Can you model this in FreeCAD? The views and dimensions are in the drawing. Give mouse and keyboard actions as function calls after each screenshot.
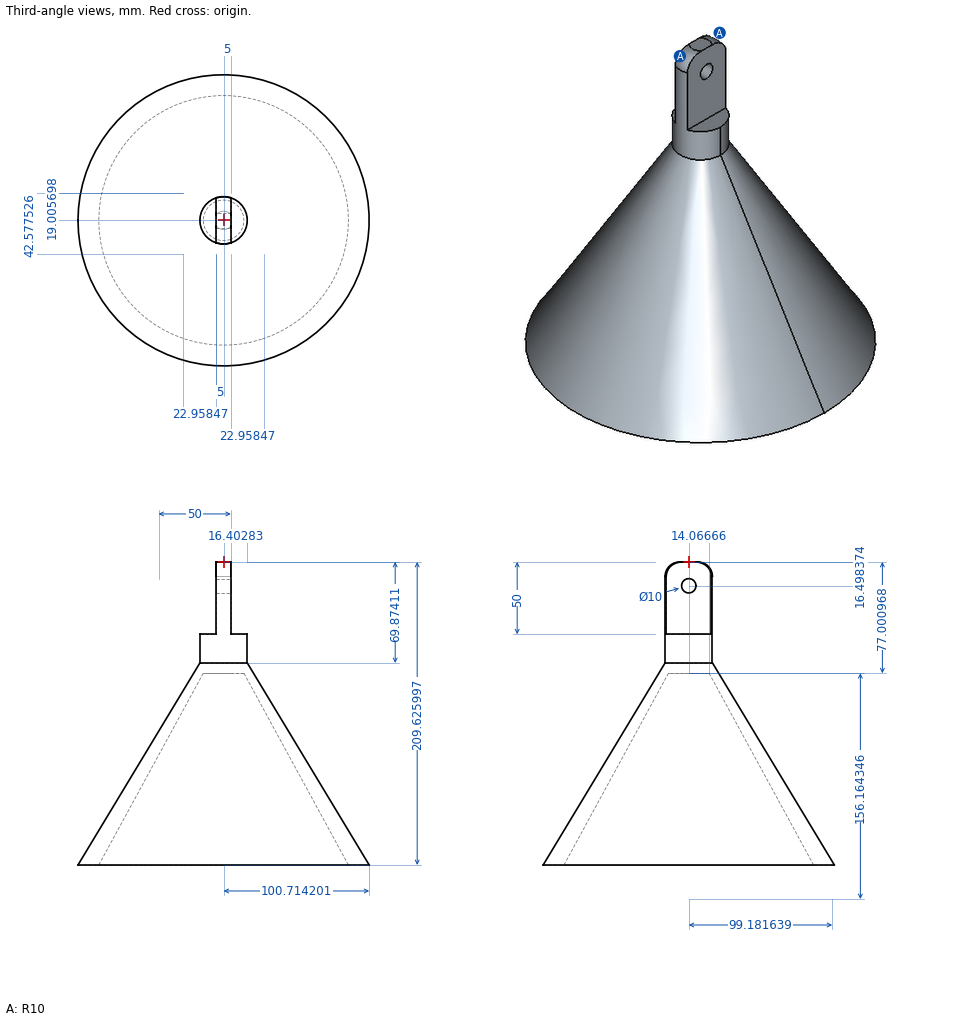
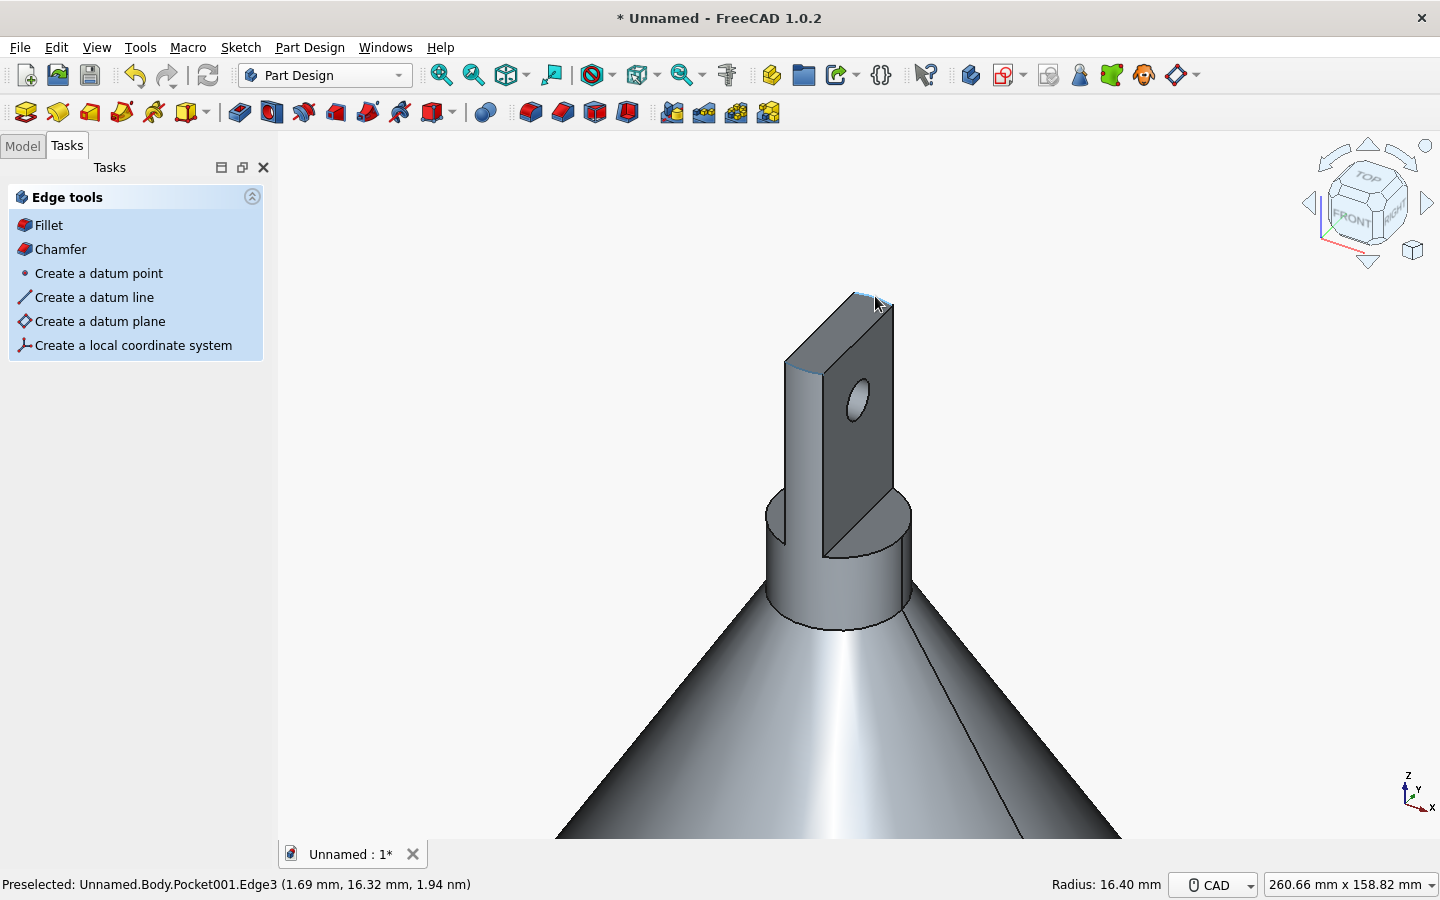
click(442, 76)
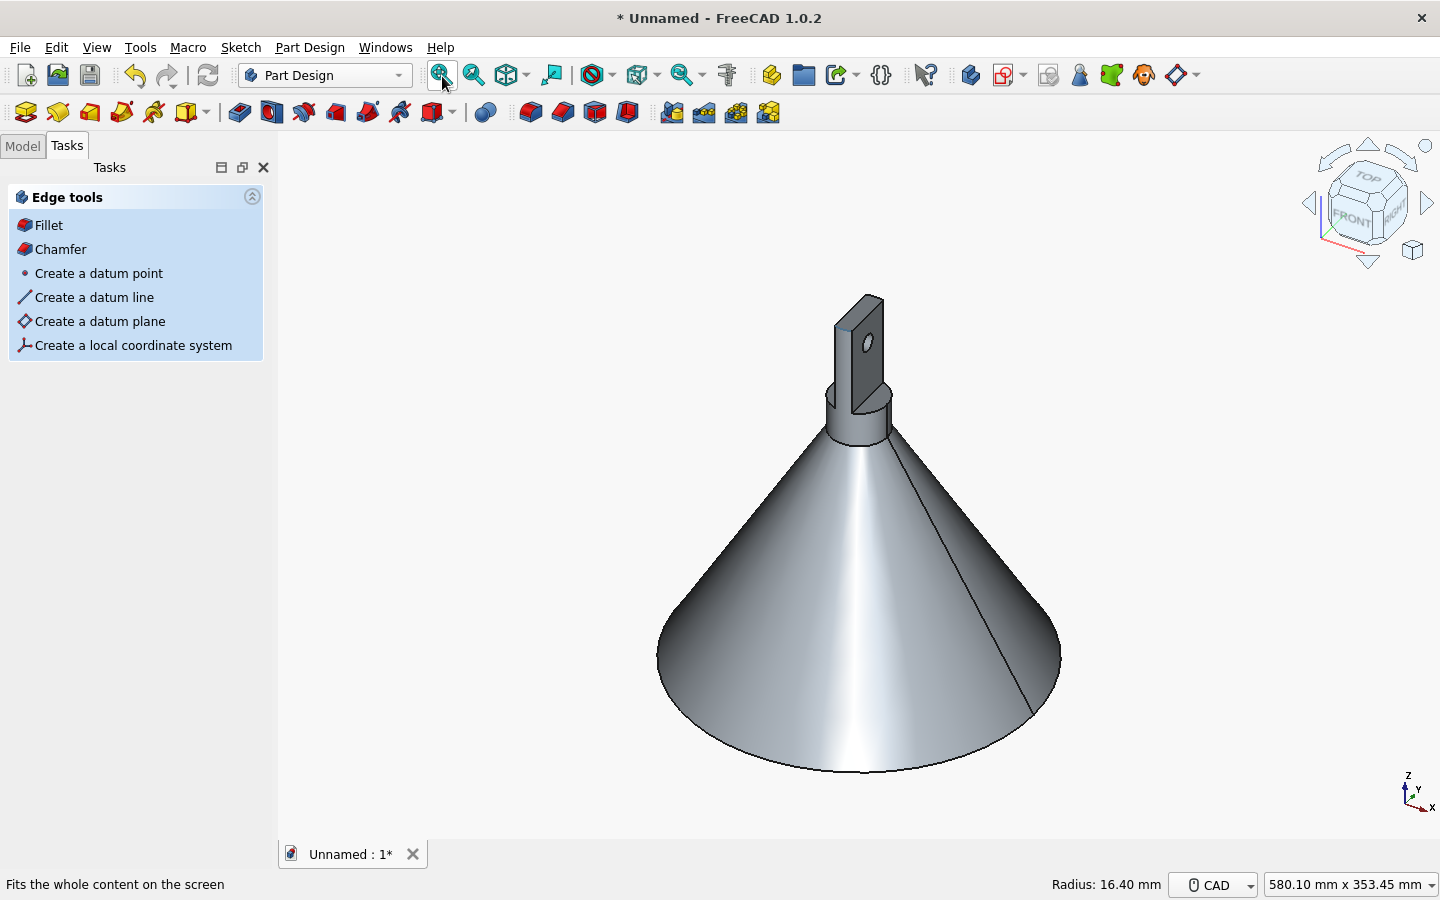
key(0)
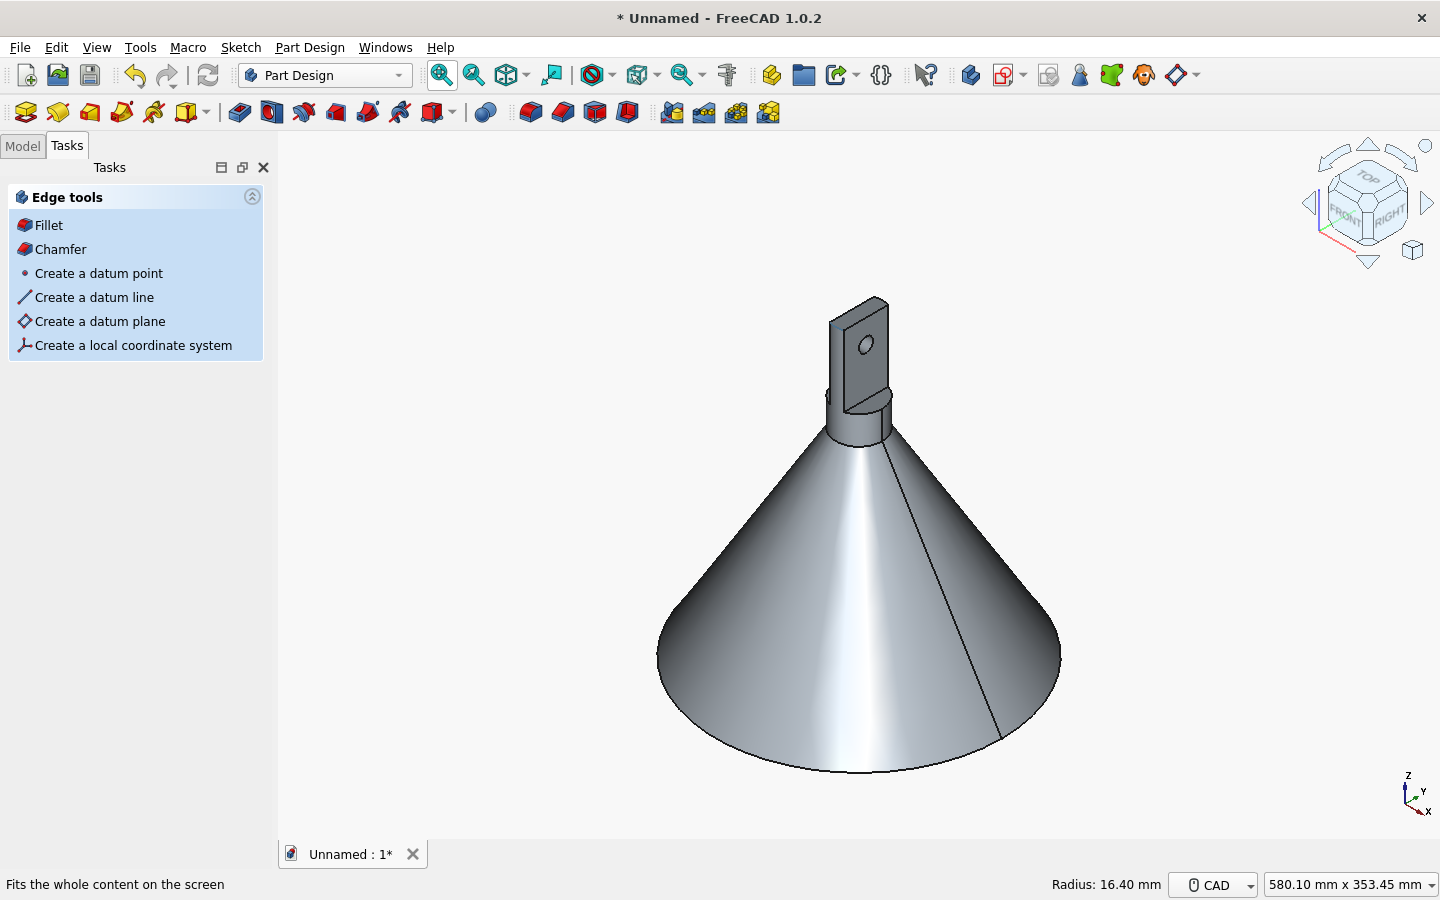
click(882, 299, ctrl)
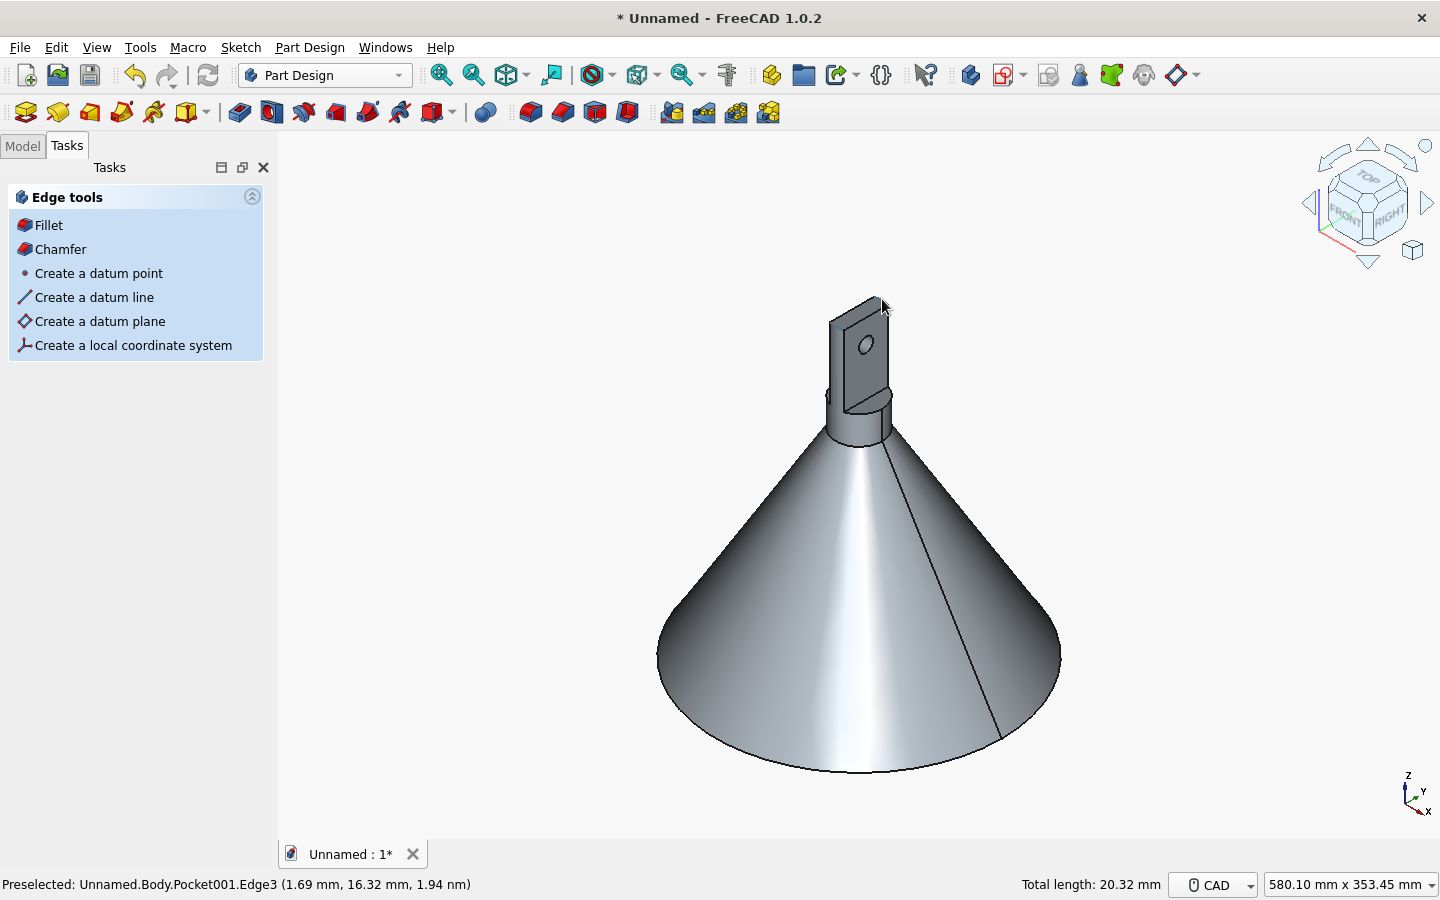
click(532, 112)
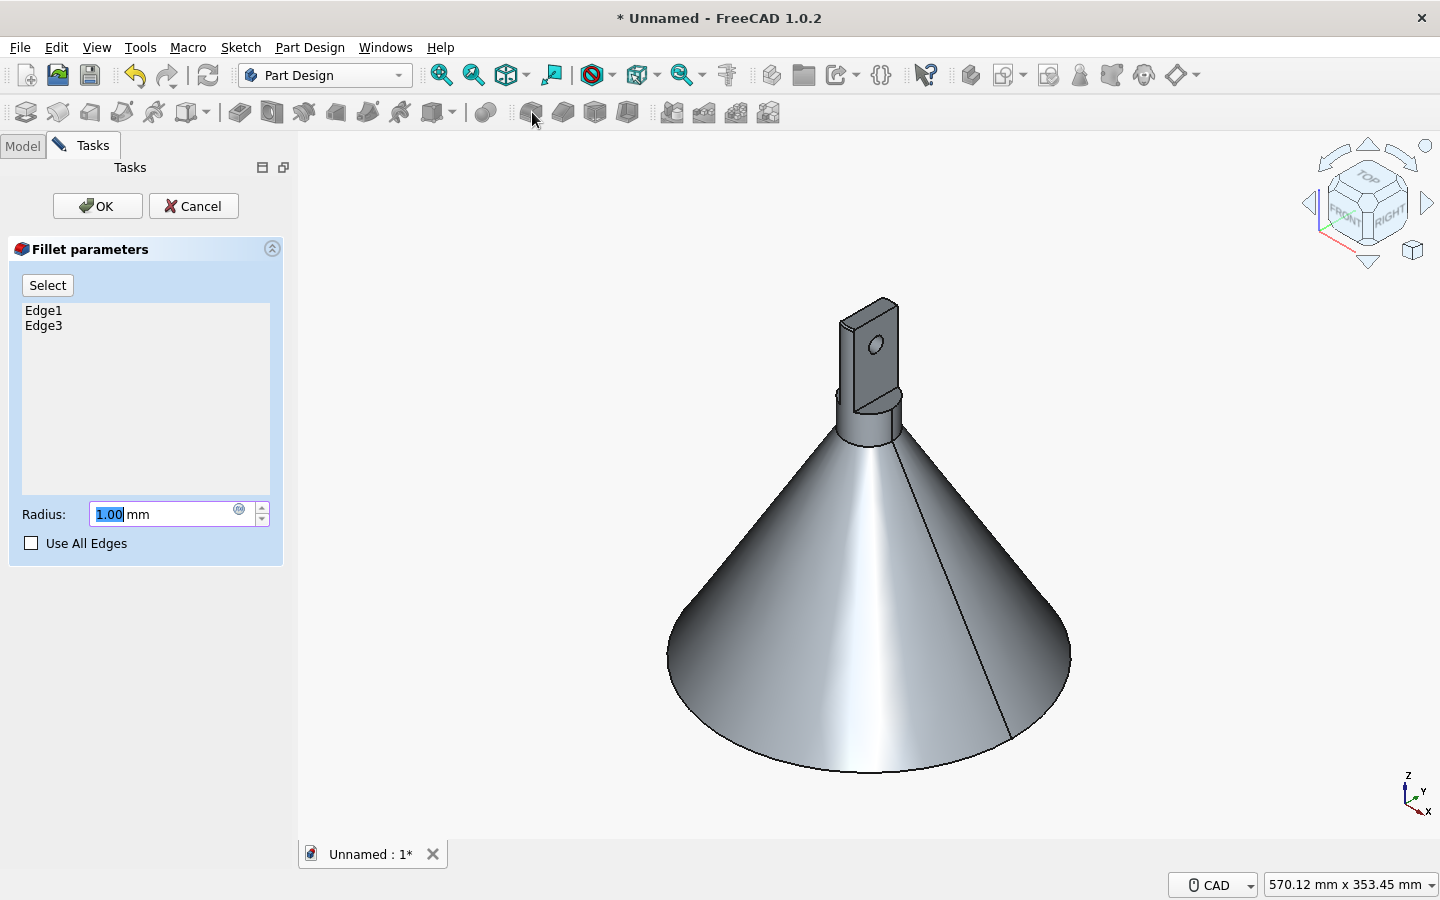
text(10)
key(Tab)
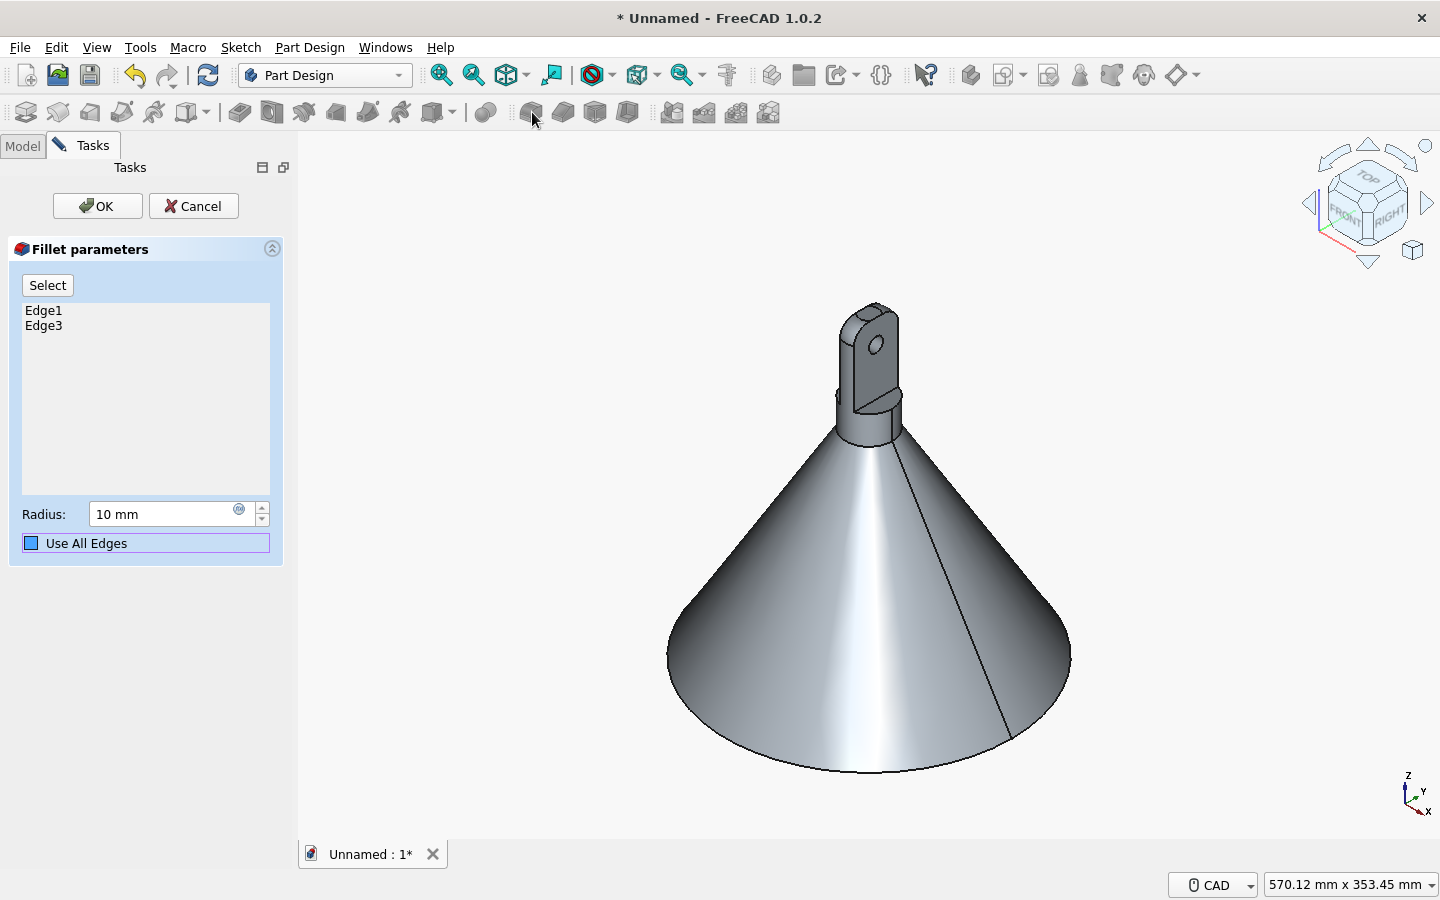
click(98, 206)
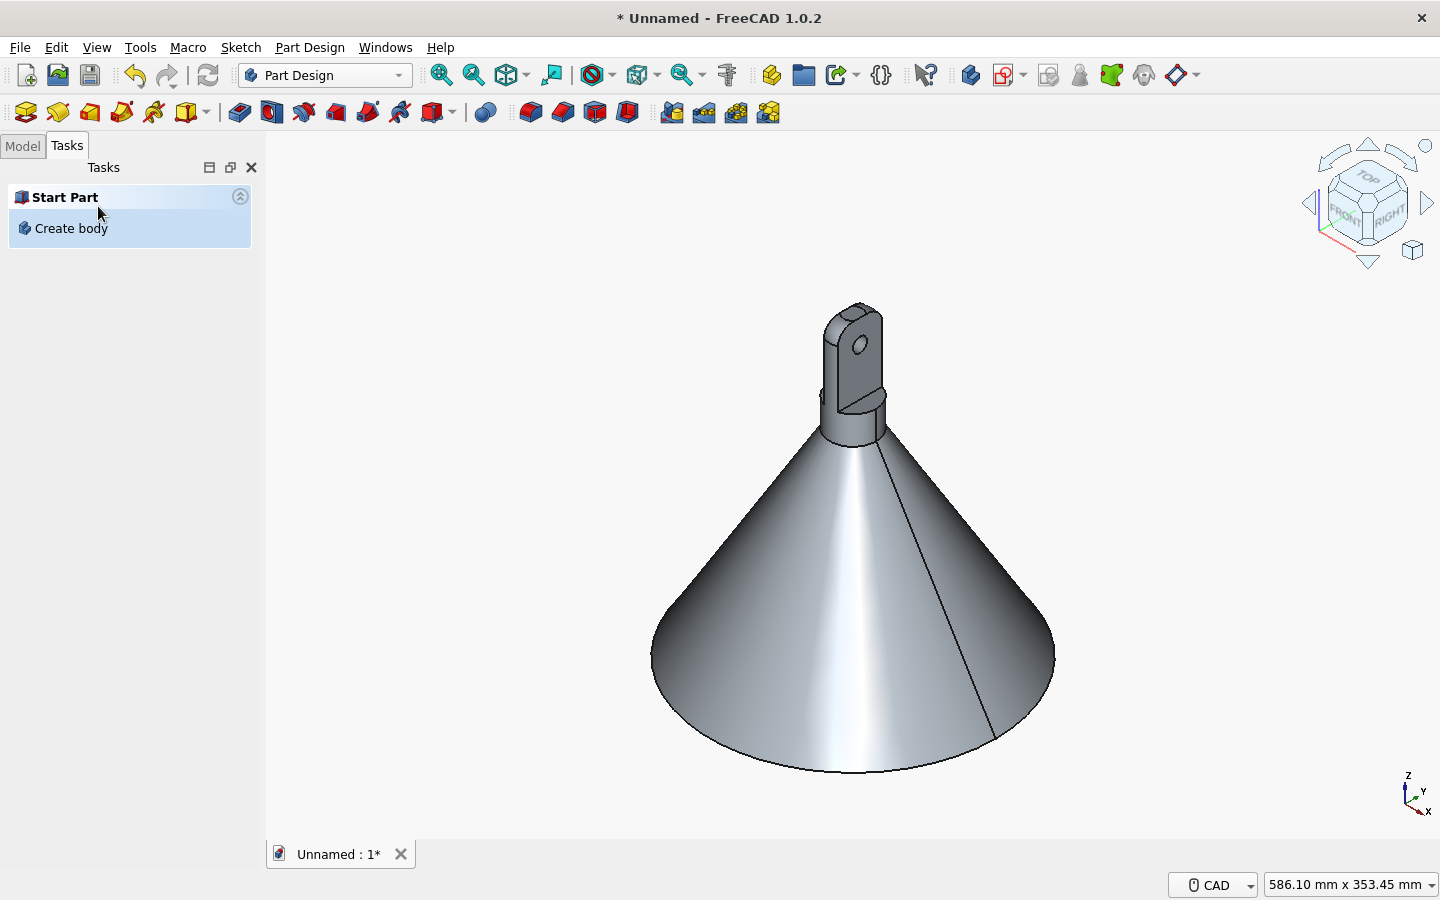
click(1004, 76)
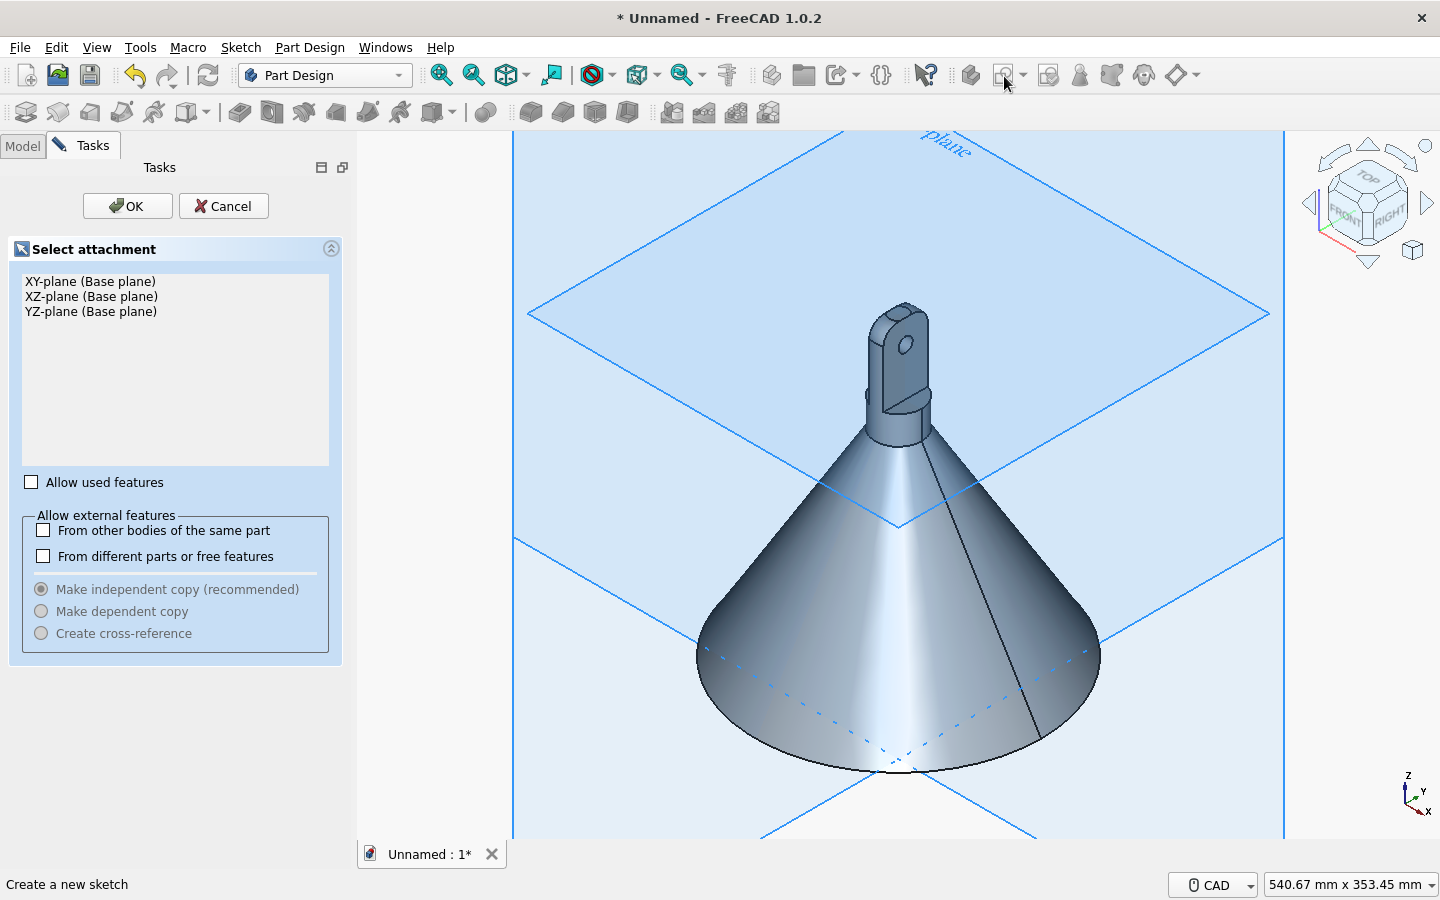
click(82, 312)